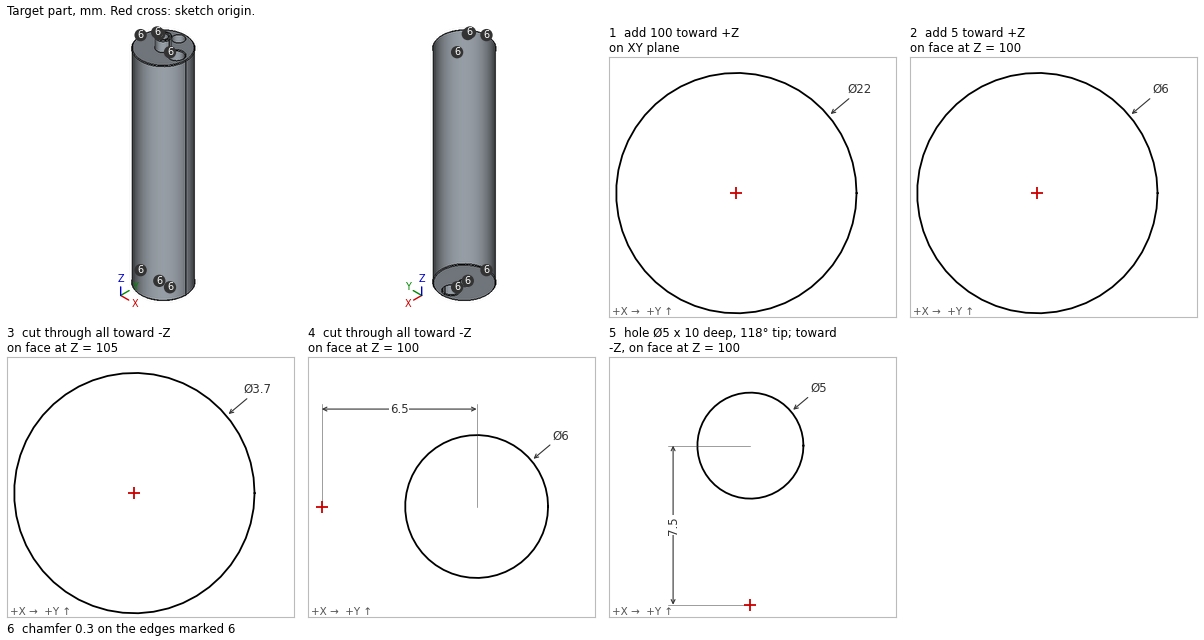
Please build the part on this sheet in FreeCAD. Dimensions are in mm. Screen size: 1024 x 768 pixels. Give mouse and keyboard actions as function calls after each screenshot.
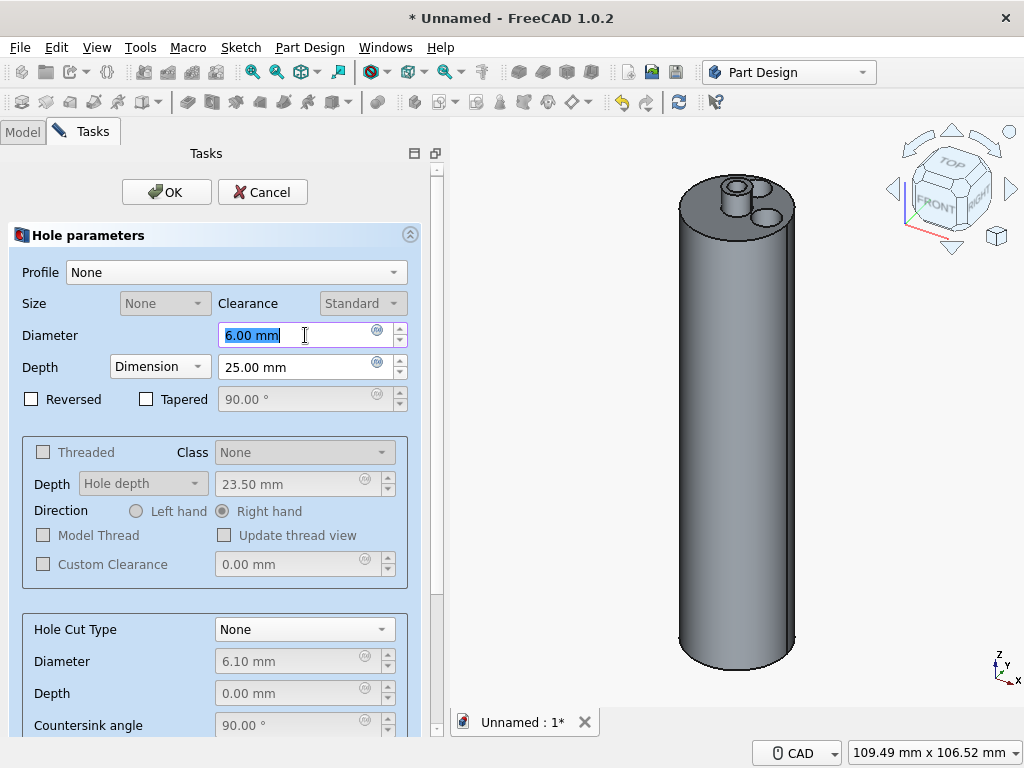
text(5)
key(Tab)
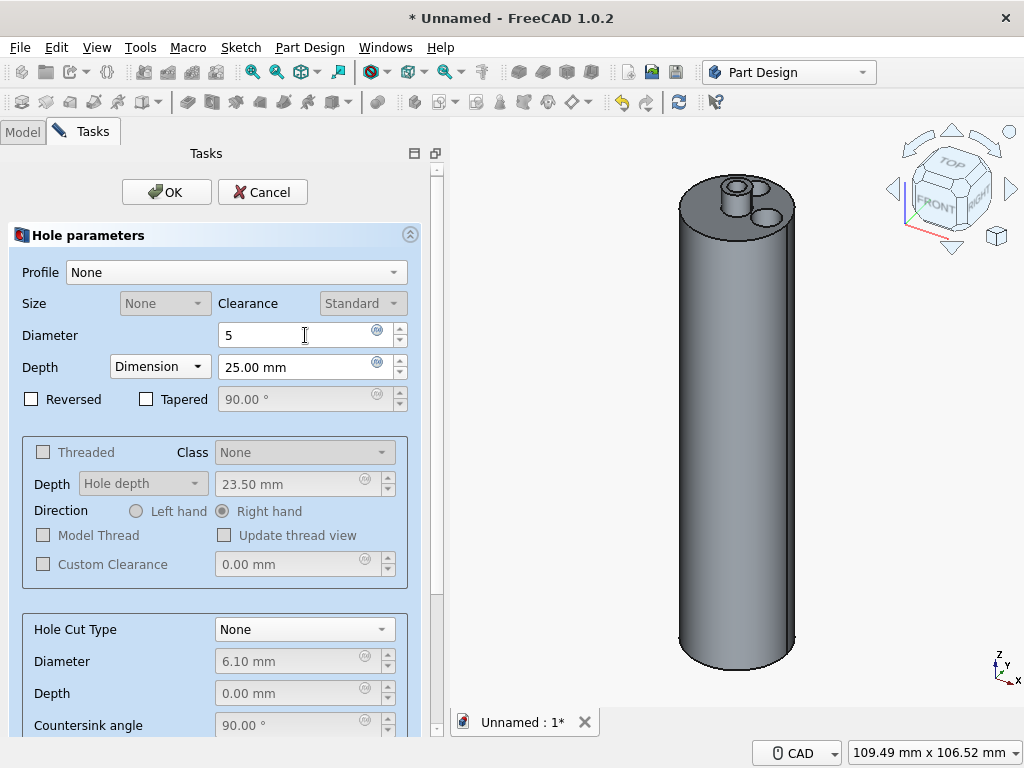
triple_click(305, 367)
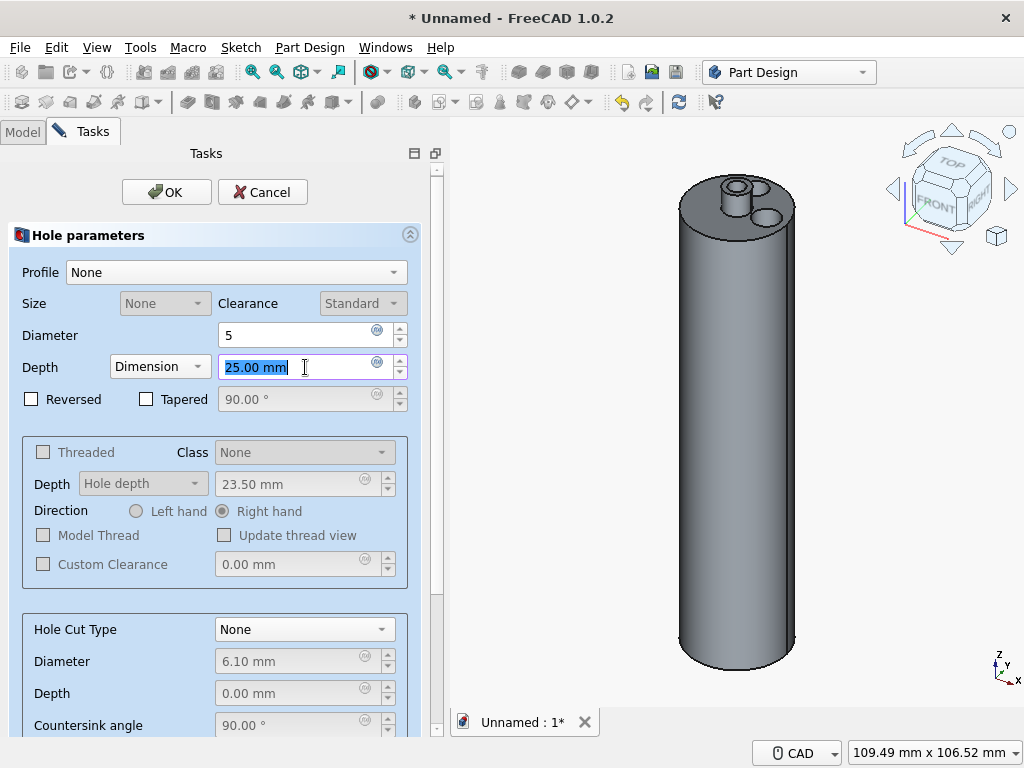
text(10)
key(Tab)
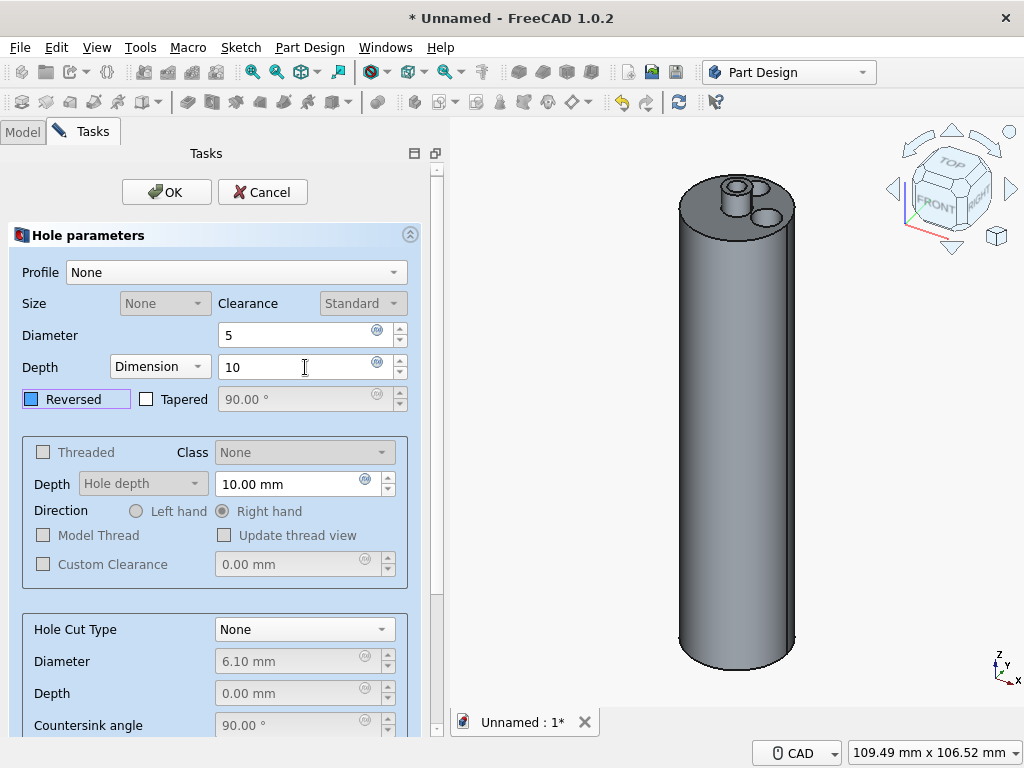
click(167, 192)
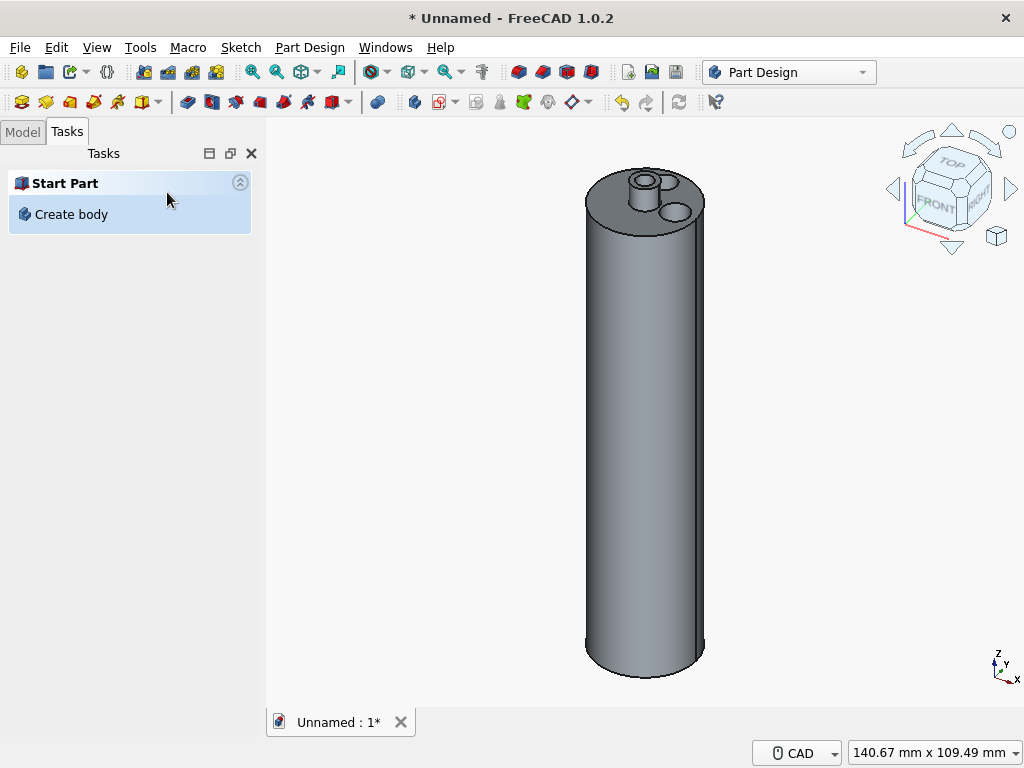
click(636, 176)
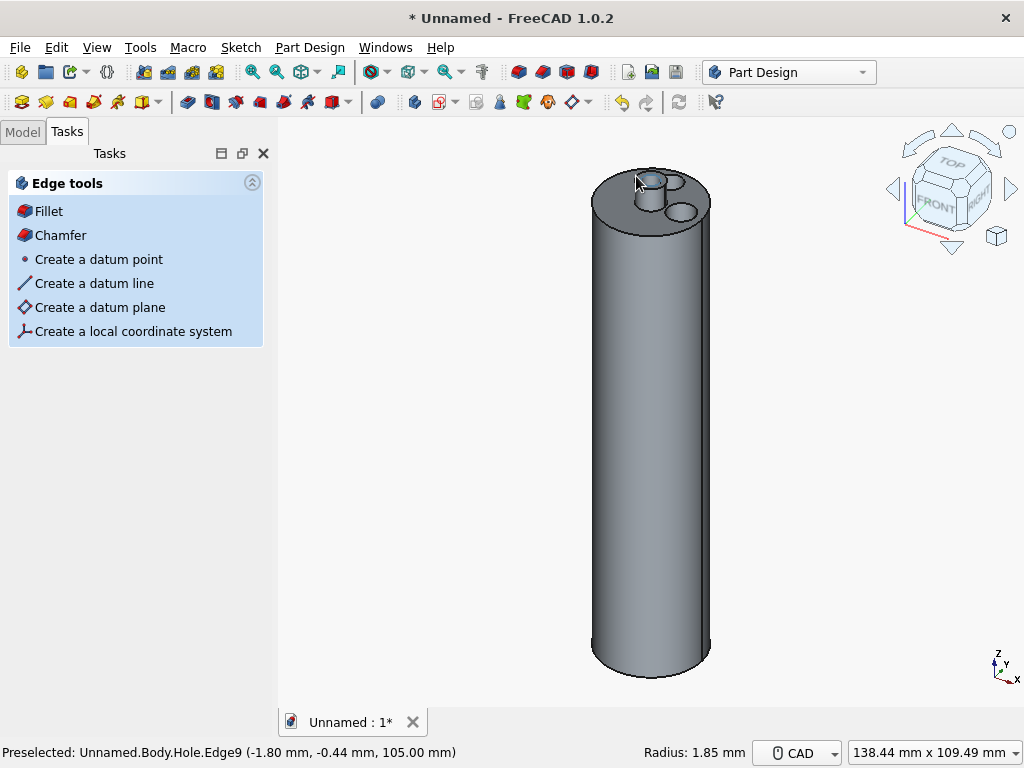
click(667, 207, ctrl)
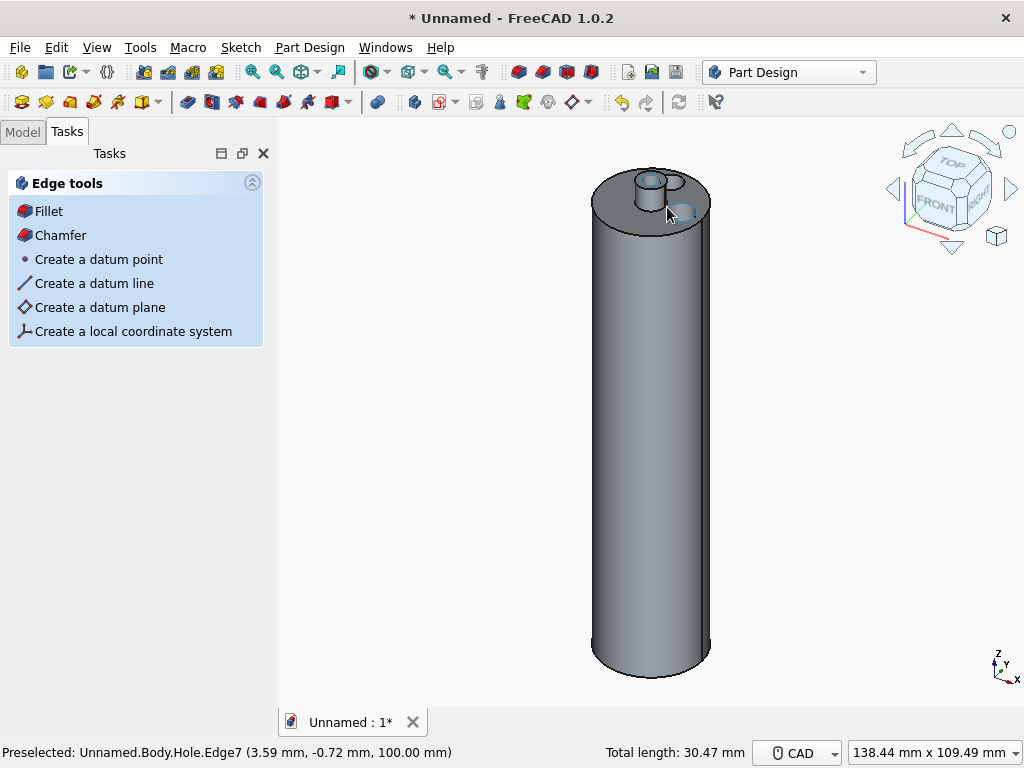
click(592, 205, ctrl)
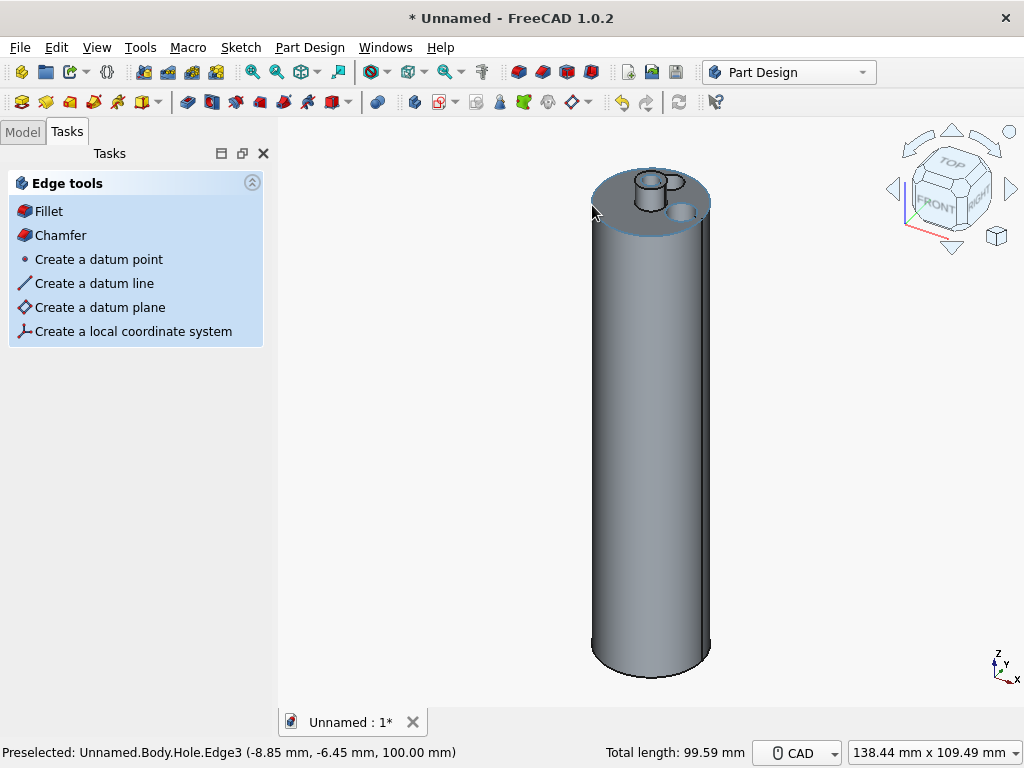
click(635, 180, ctrl)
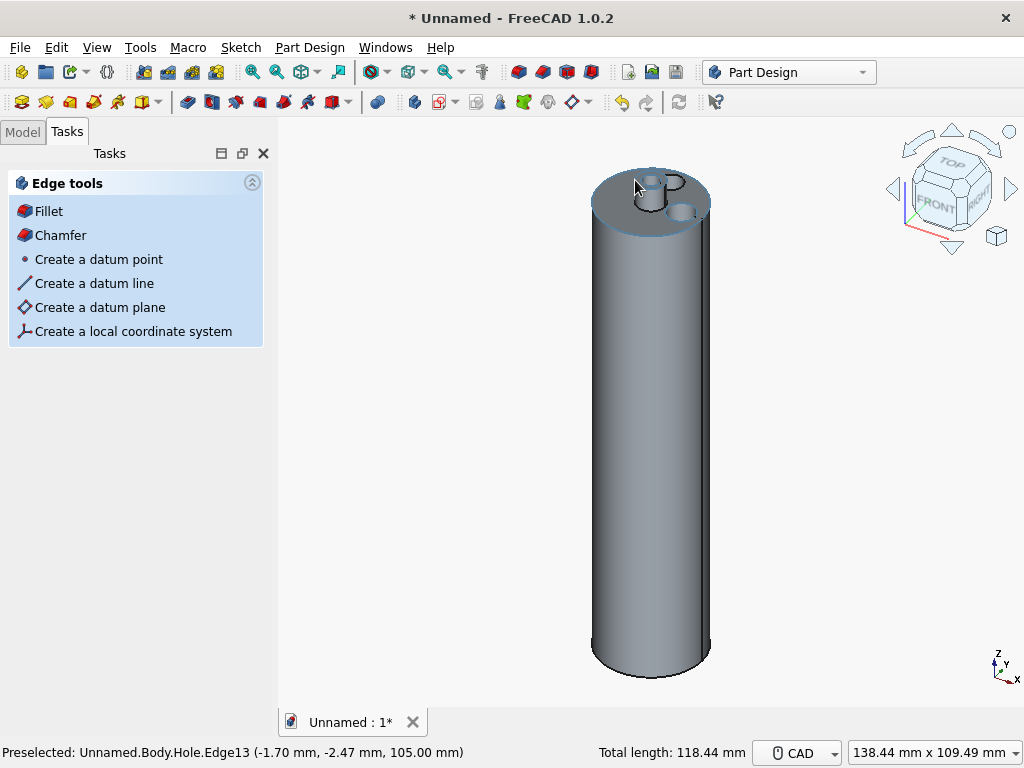
key(0)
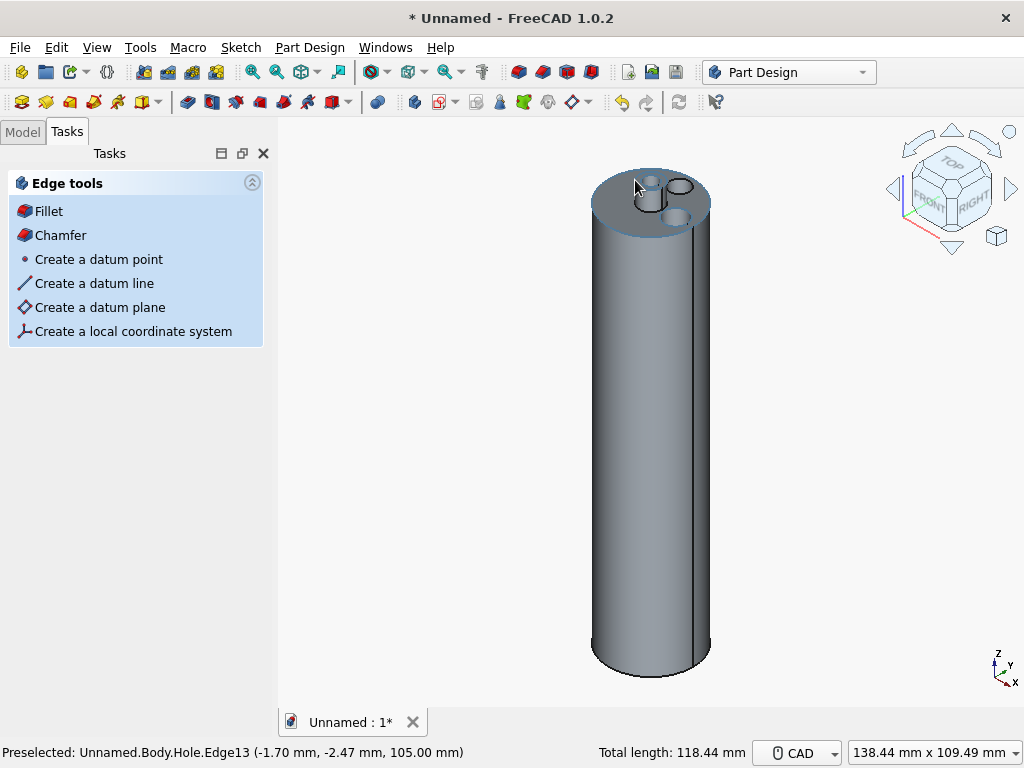
key(2)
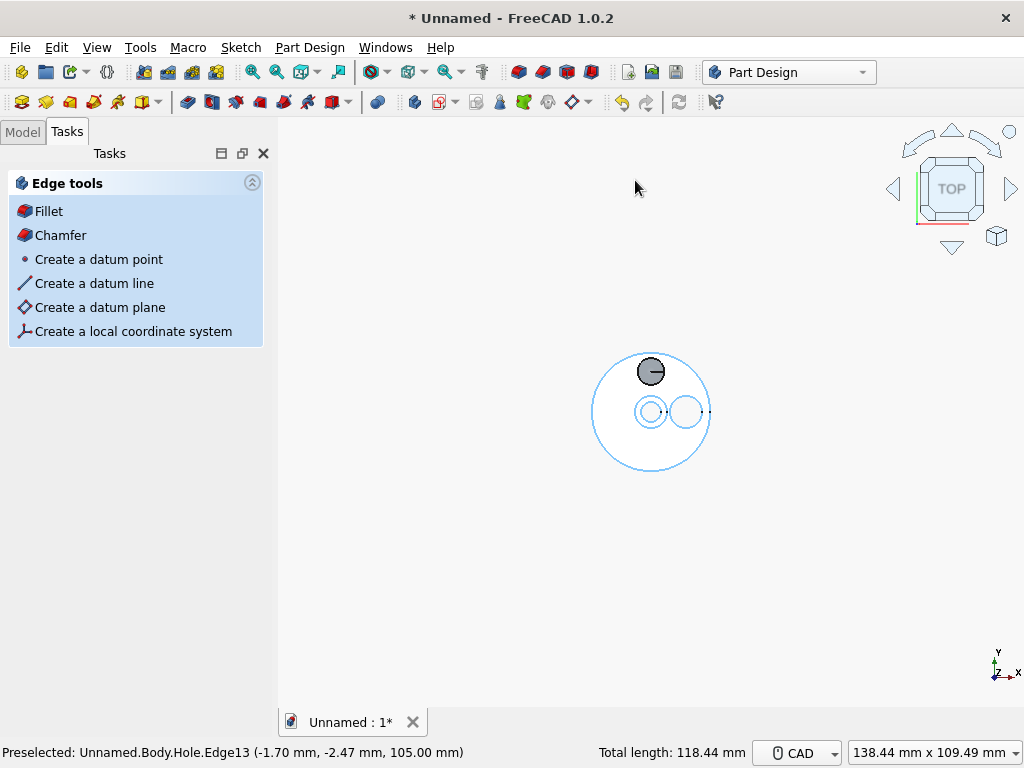
key(v)
key(f)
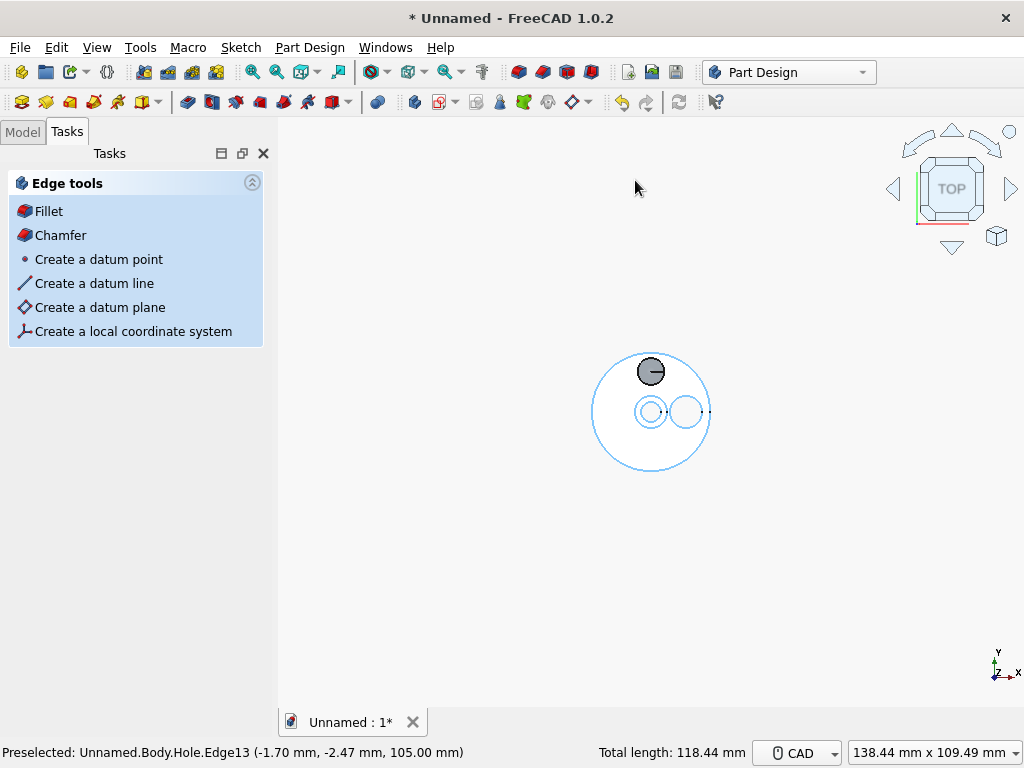
key(1)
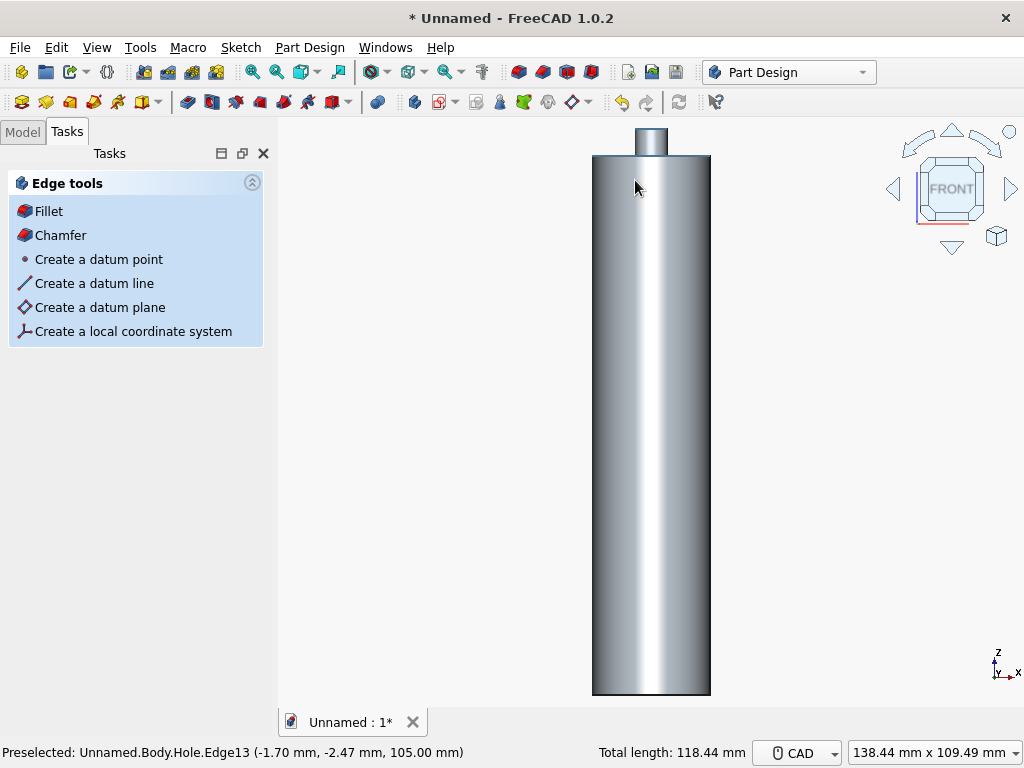
key(3)